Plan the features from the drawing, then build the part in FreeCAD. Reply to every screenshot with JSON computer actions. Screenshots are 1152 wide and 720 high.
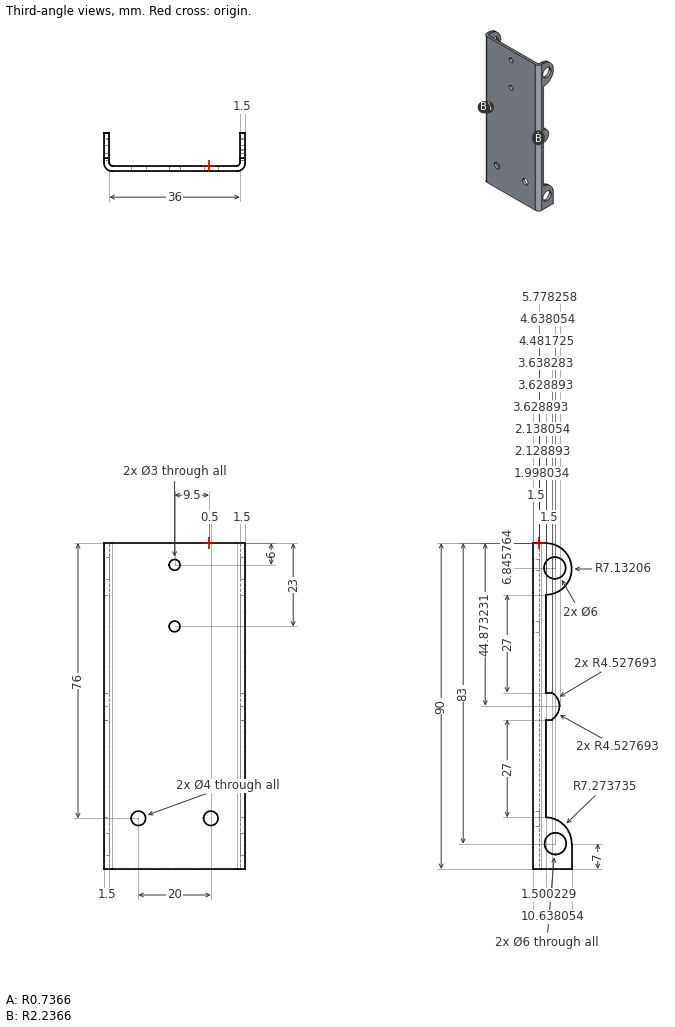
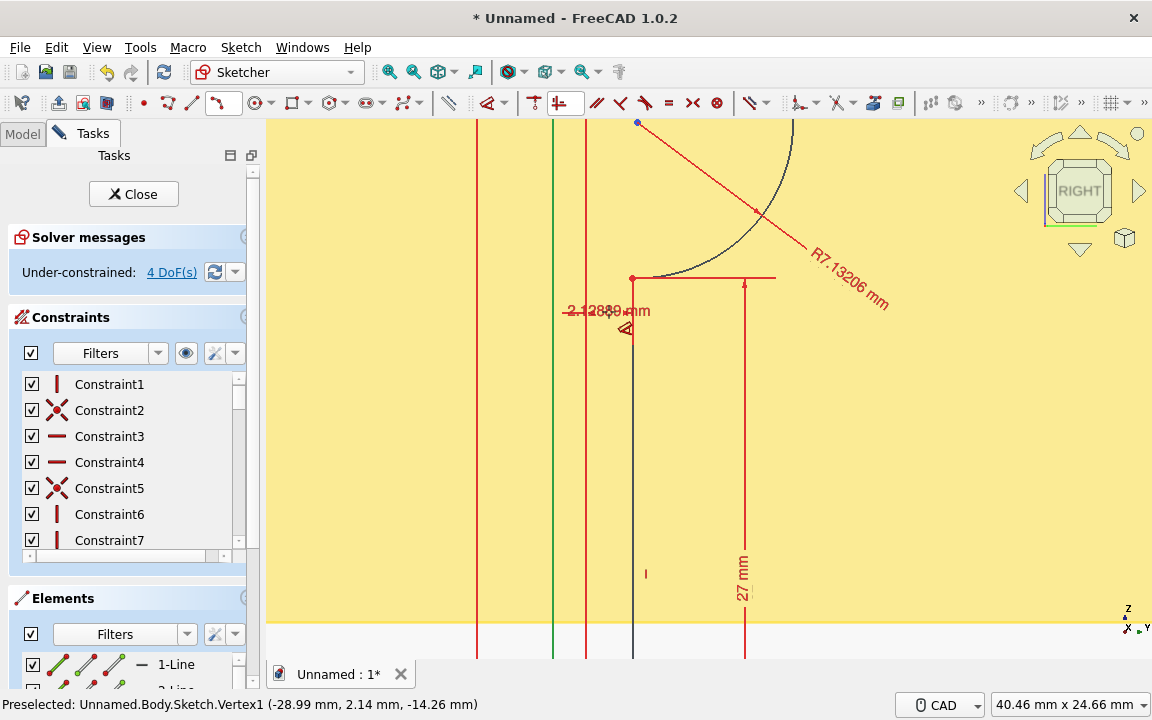
{"action": "scroll", "coordinate": [635, 278], "scroll_direction": "down", "scroll_amount": 9}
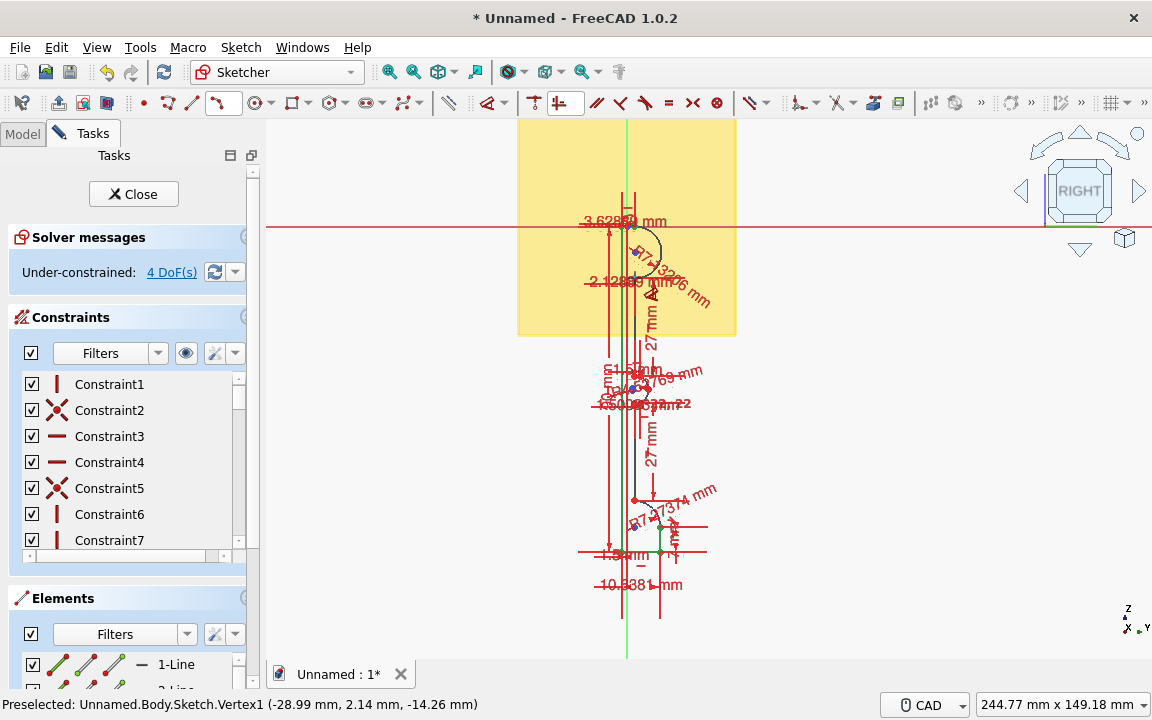
{"action": "scroll", "coordinate": [640, 403], "scroll_direction": "up", "scroll_amount": 6}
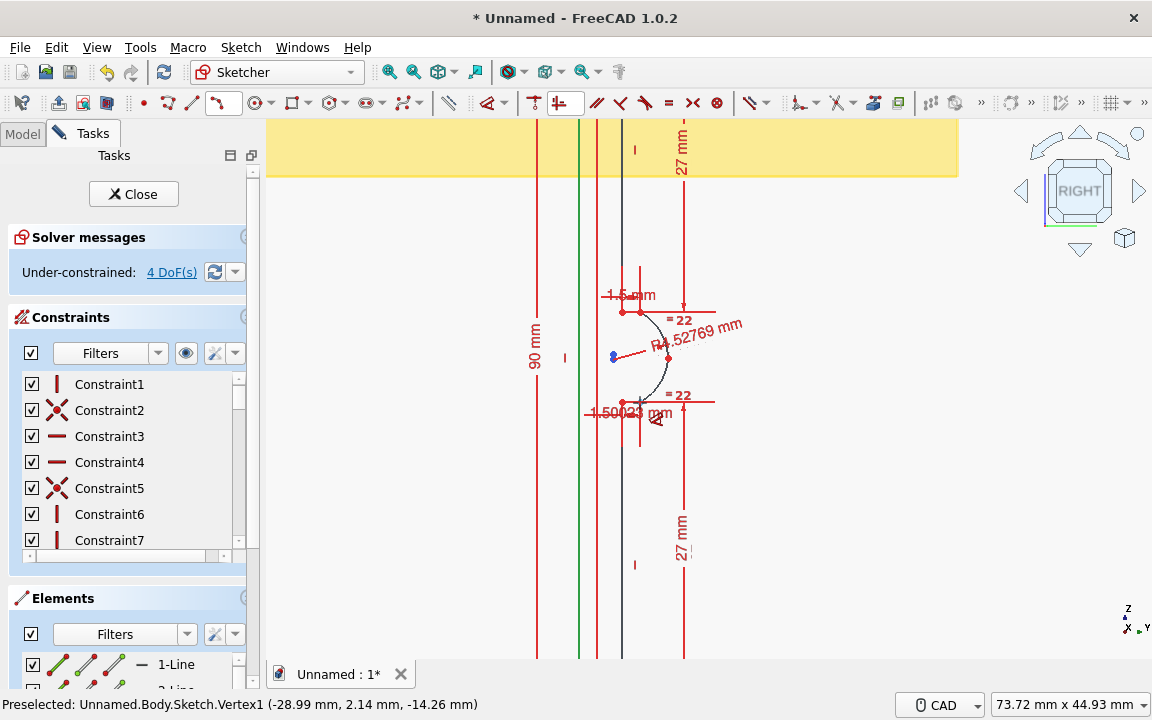
{"action": "left_click", "coordinate": [640, 402]}
{"action": "left_click", "coordinate": [608, 436]}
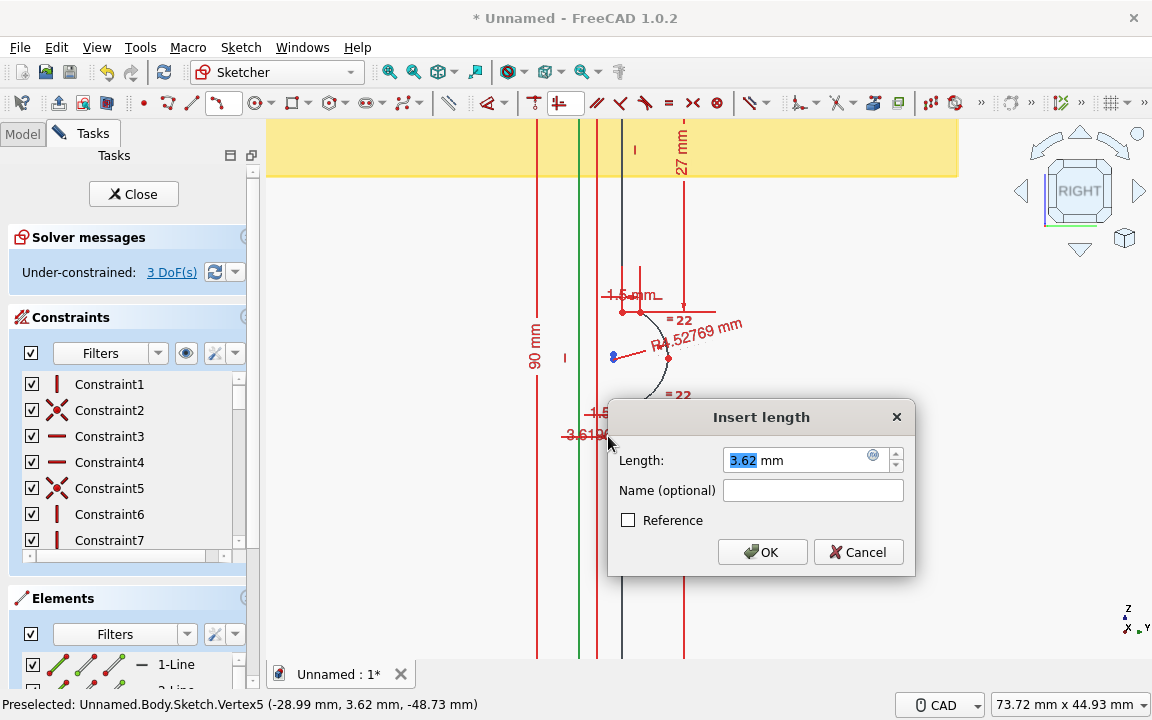
{"action": "type", "text": "3.638283"}
{"action": "key", "text": "Return"}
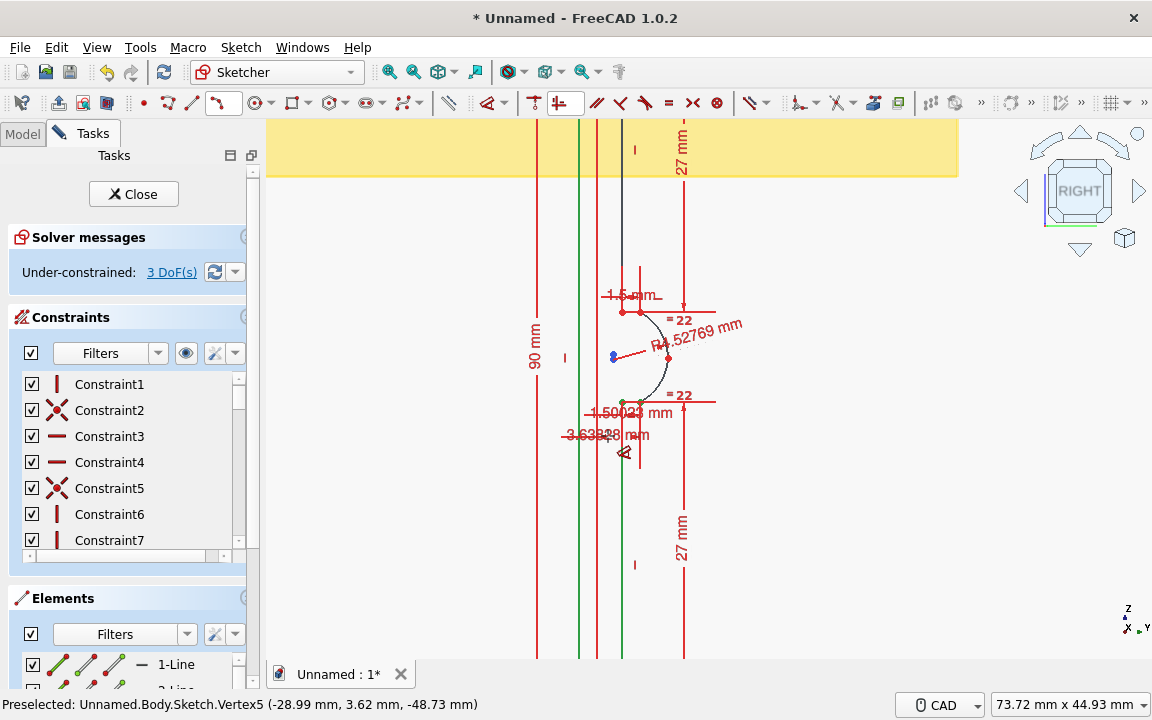
{"action": "left_click", "coordinate": [668, 358]}
{"action": "left_click", "coordinate": [649, 464]}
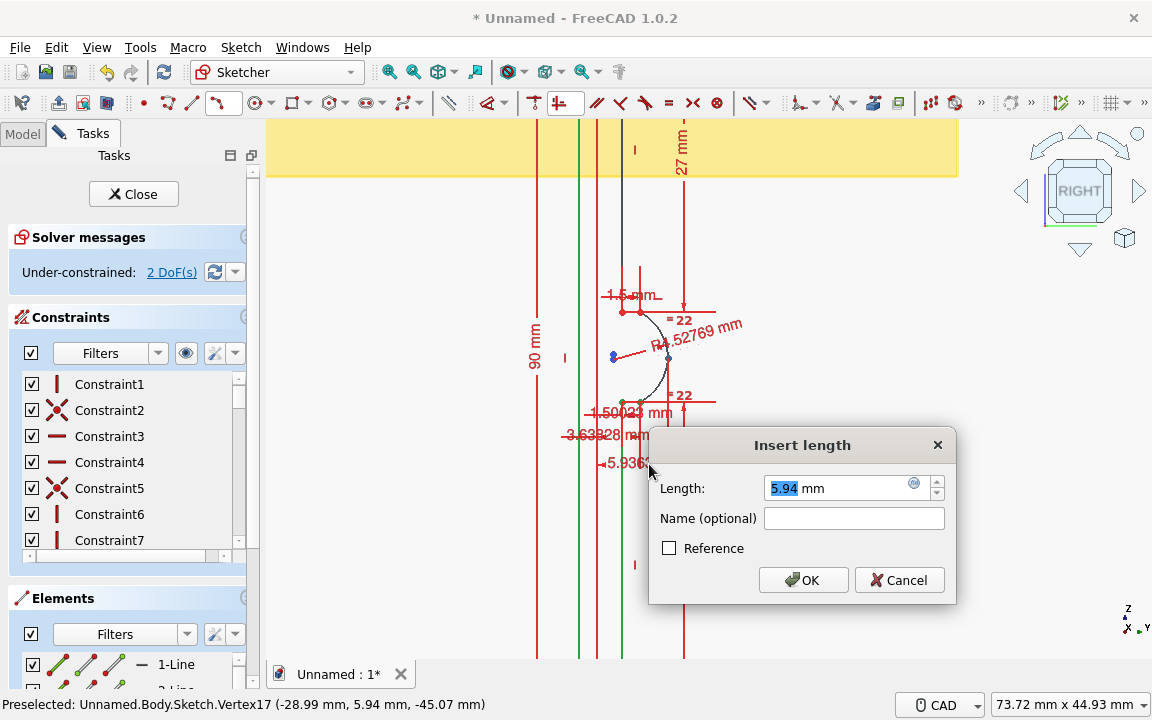
{"action": "type", "text": "5.778258"}
{"action": "key", "text": "Return"}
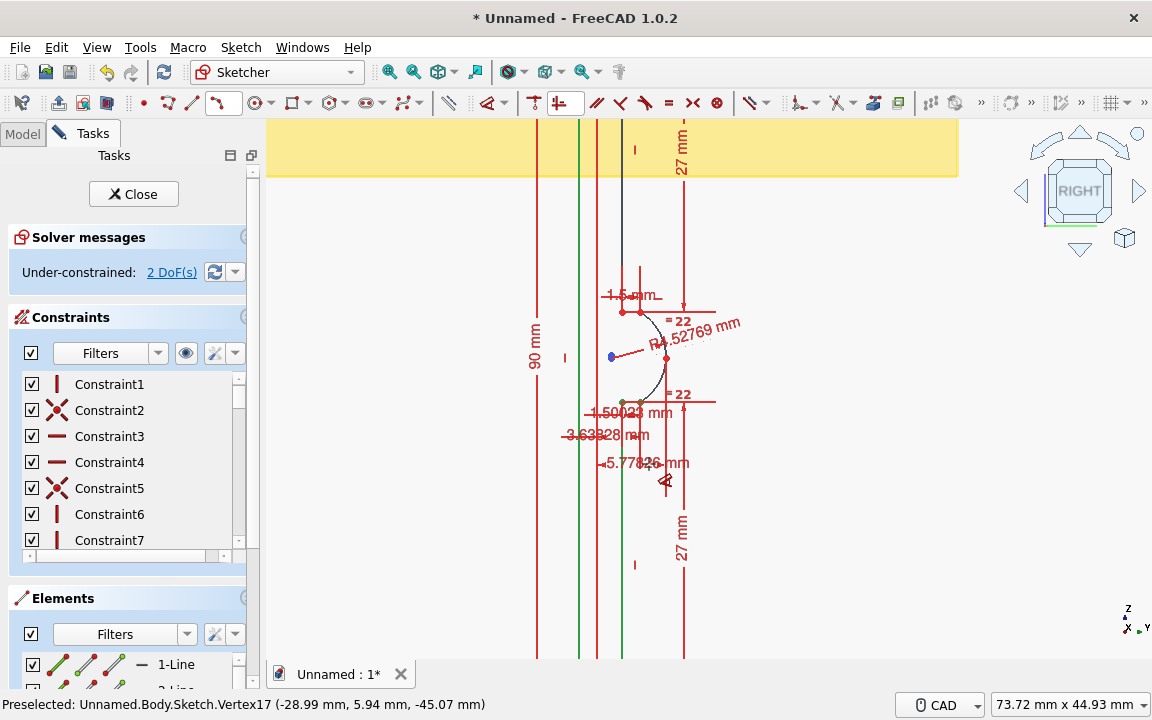
{"action": "scroll", "coordinate": [640, 403], "scroll_direction": "down", "scroll_amount": 6}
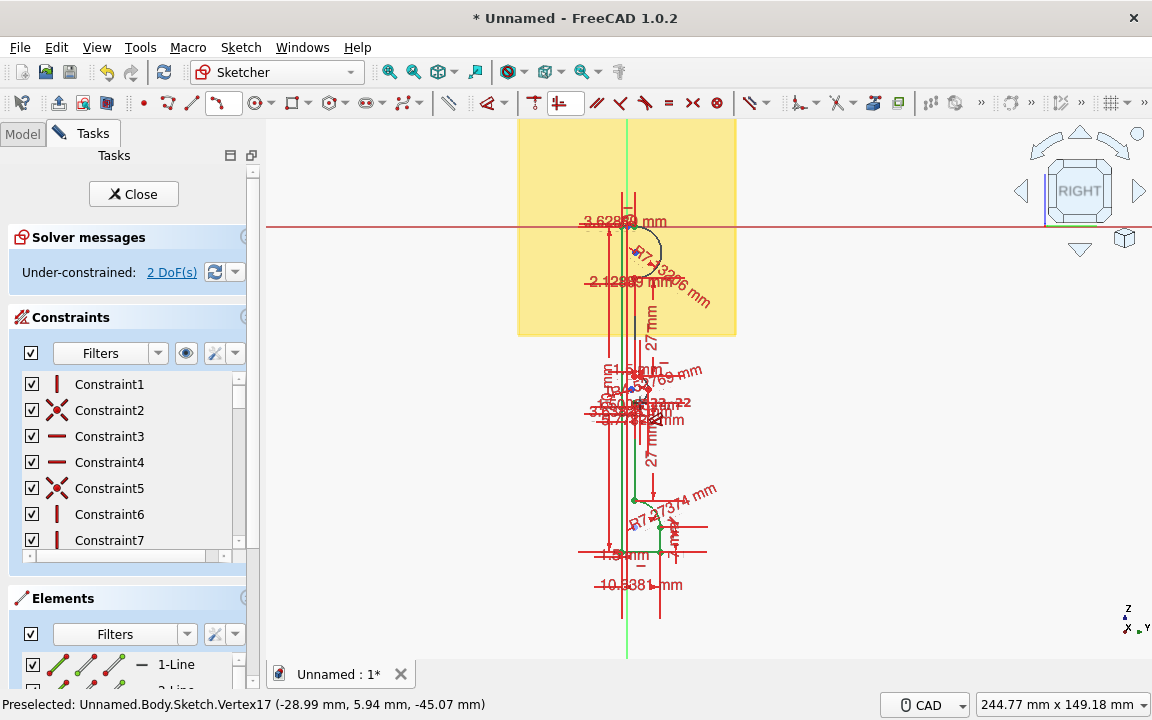
{"action": "scroll", "coordinate": [636, 252], "scroll_direction": "up", "scroll_amount": 9}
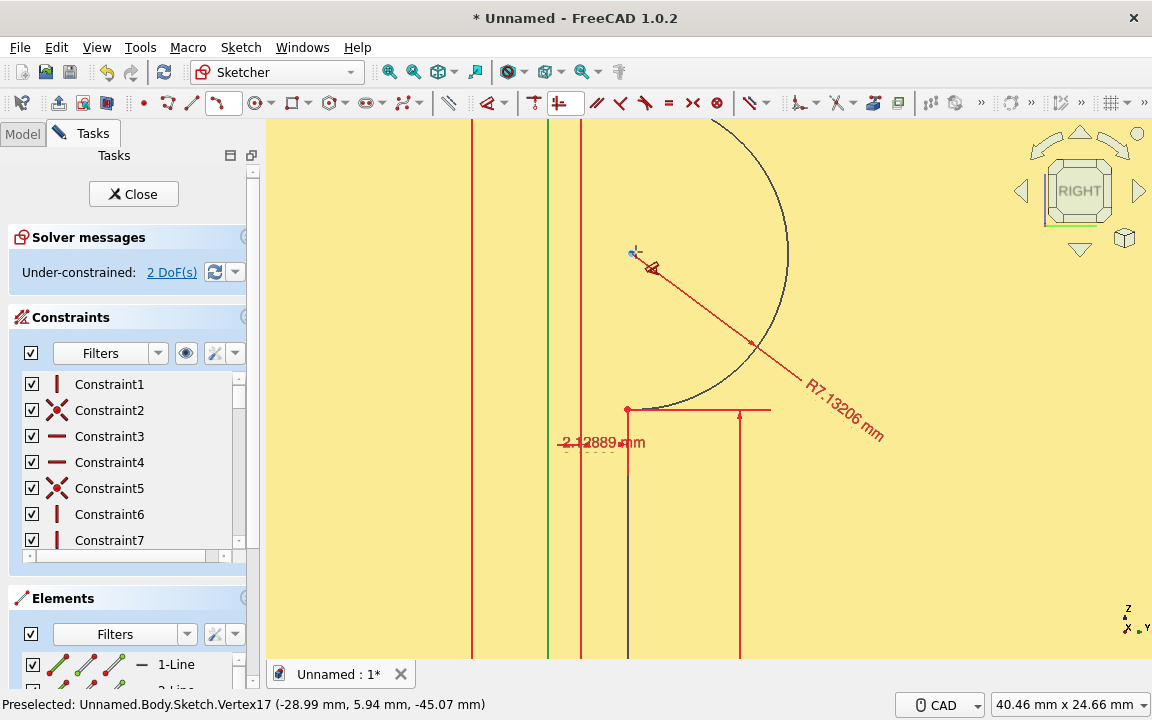
{"action": "left_click", "coordinate": [632, 254]}
{"action": "left_click", "coordinate": [606, 288]}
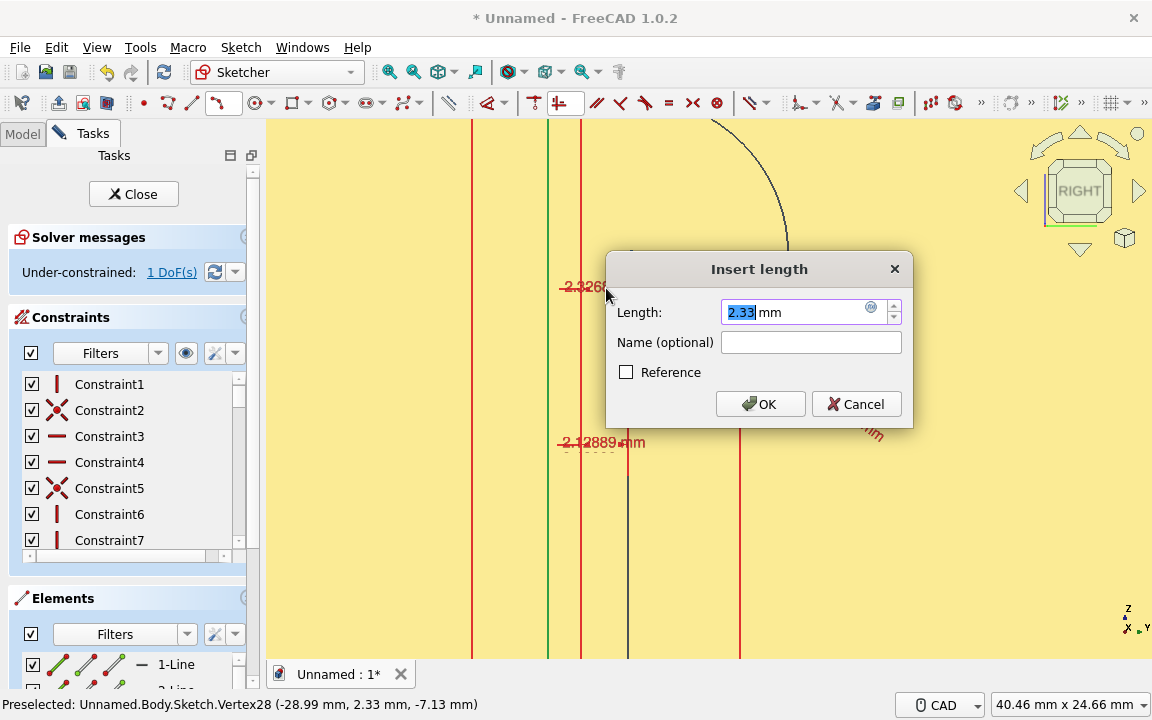
{"action": "type", "text": "1.998034"}
{"action": "key", "text": "Return"}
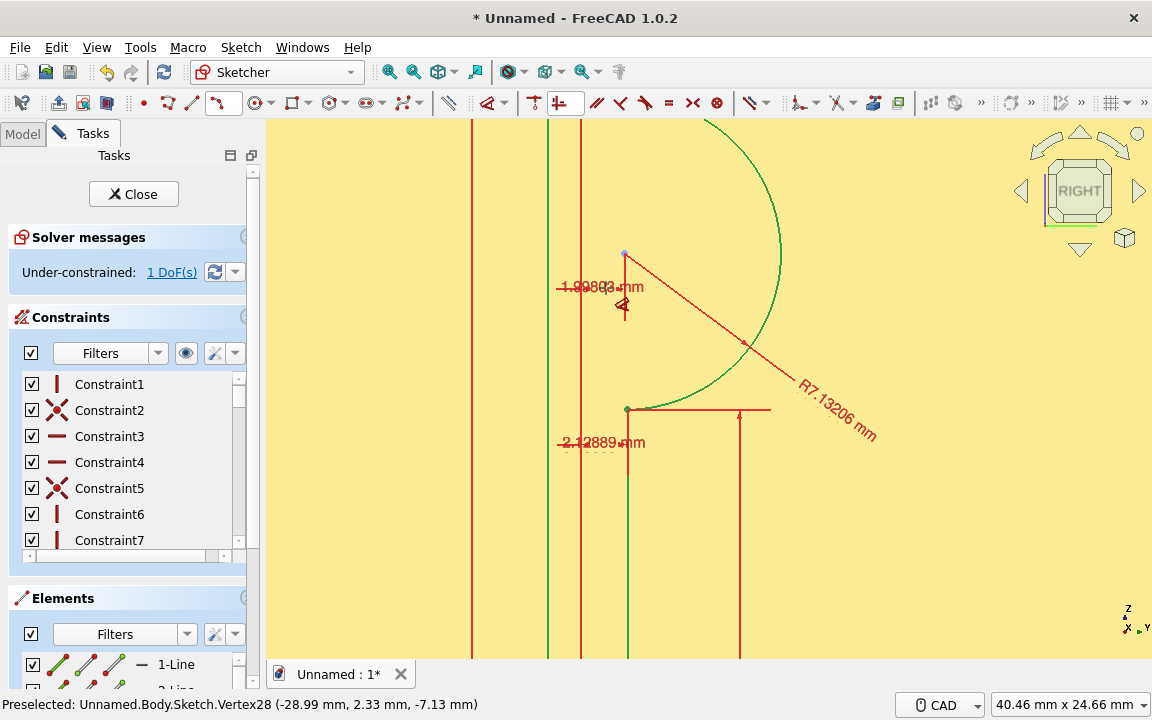
{"action": "scroll", "coordinate": [636, 252], "scroll_direction": "down", "scroll_amount": 9}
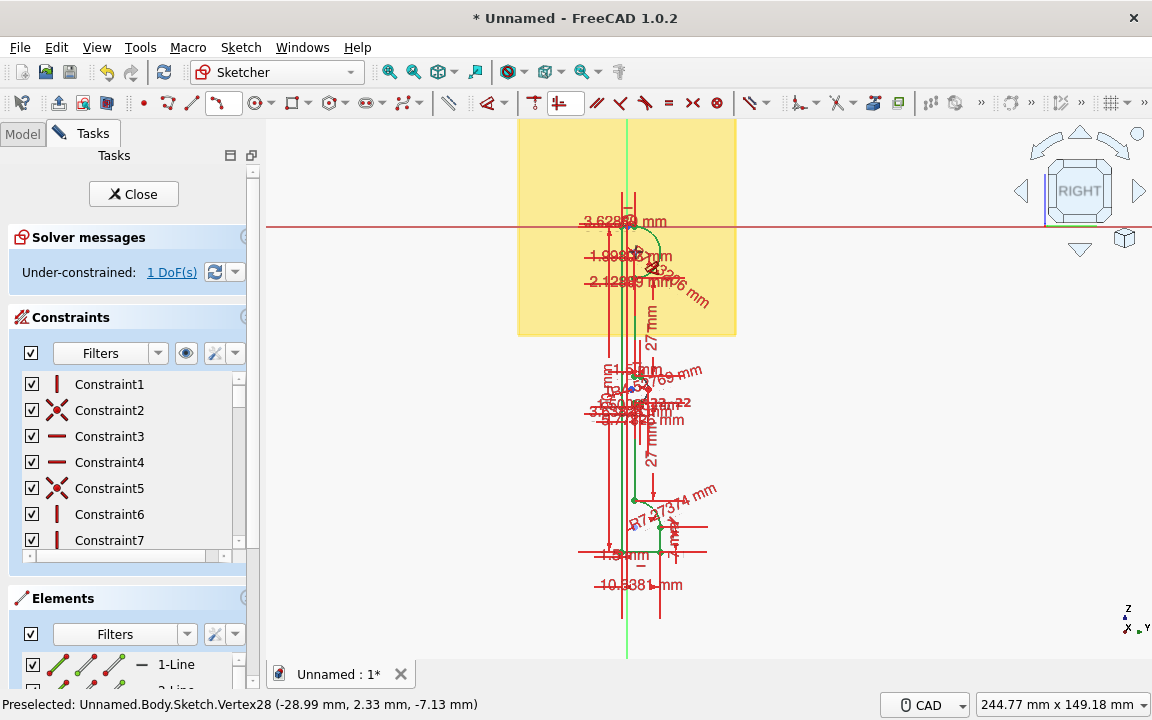
{"action": "left_click", "coordinate": [648, 390]}
{"action": "left_click", "coordinate": [569, 308]}